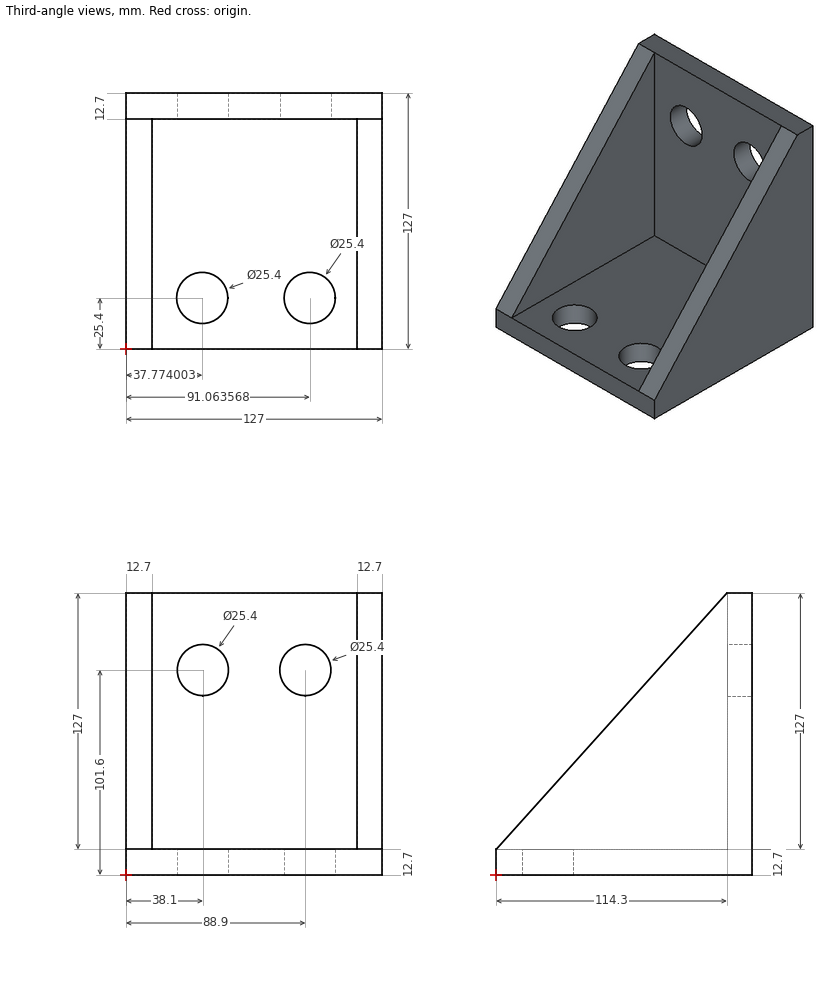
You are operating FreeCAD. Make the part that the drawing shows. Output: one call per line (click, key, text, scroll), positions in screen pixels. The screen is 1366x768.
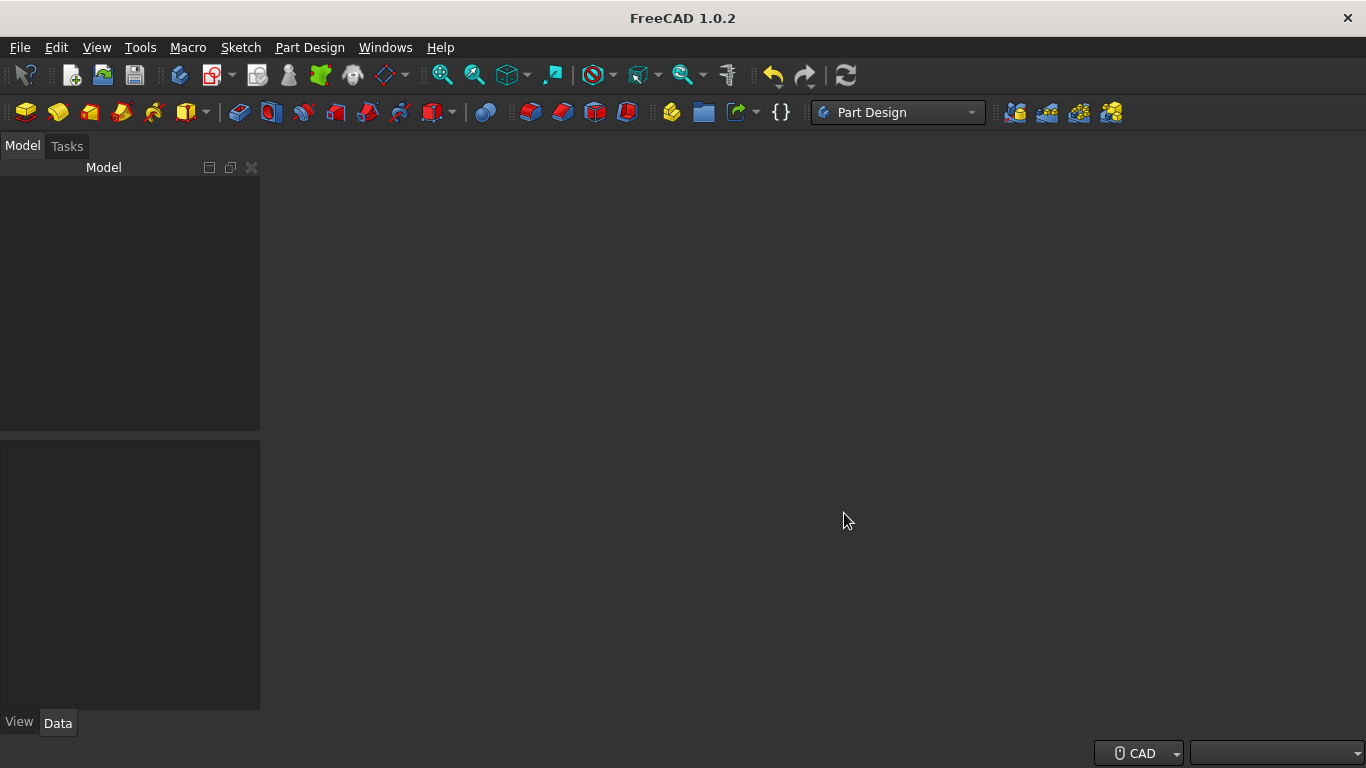
key(ctrl+n)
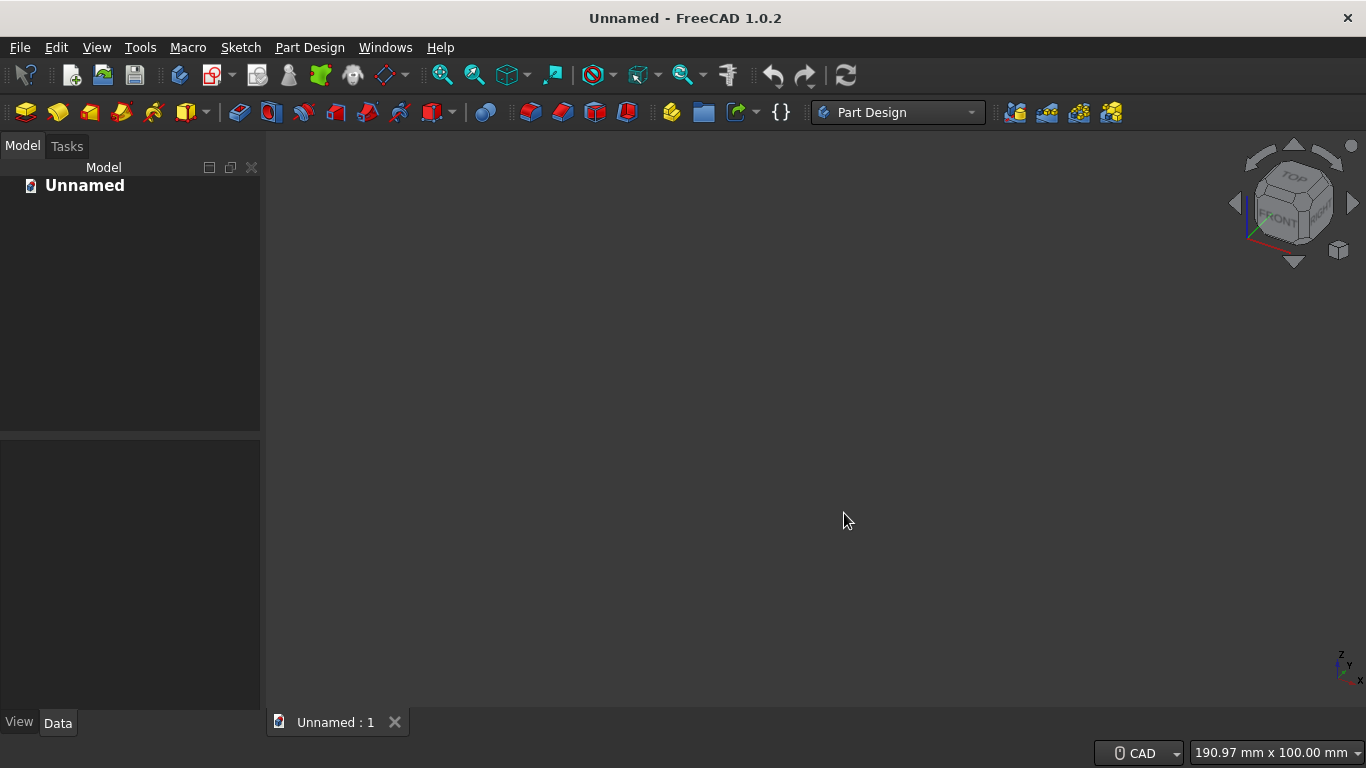
click(212, 76)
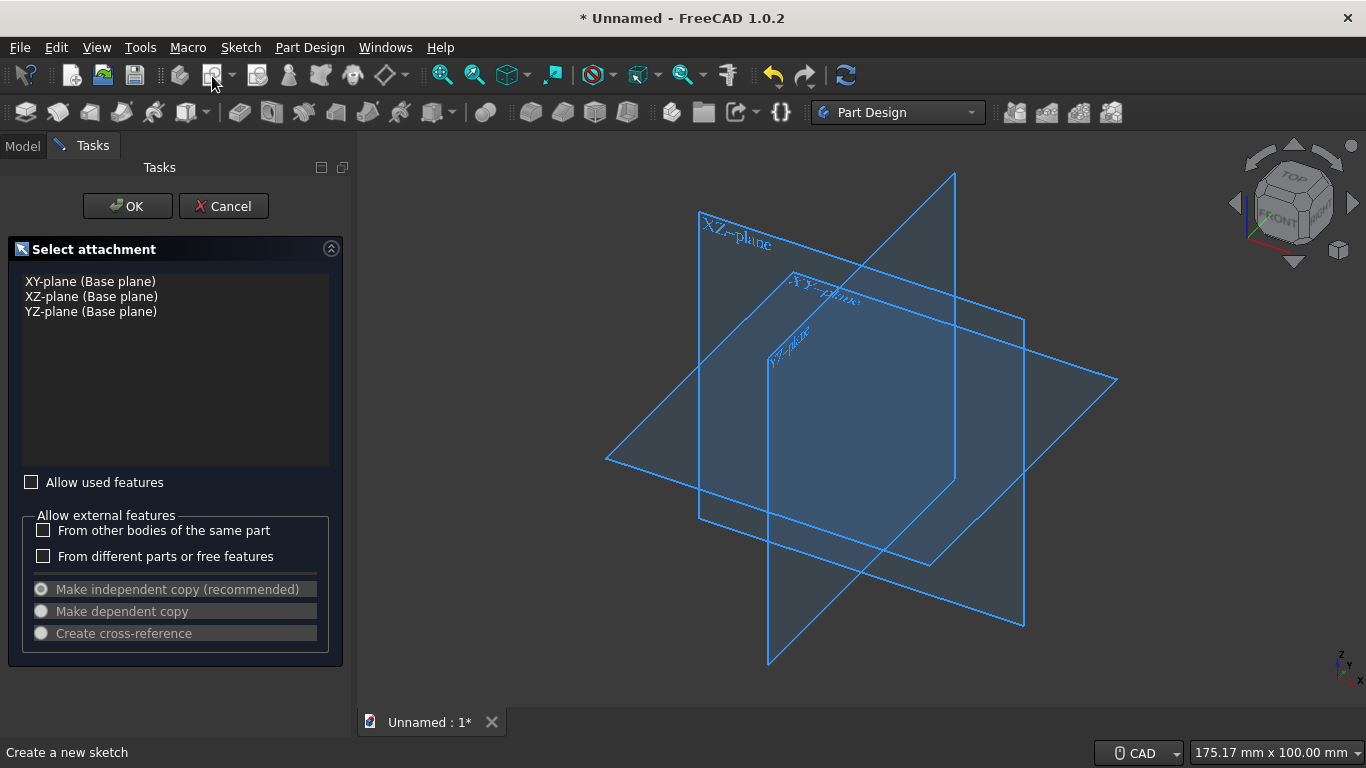
click(82, 282)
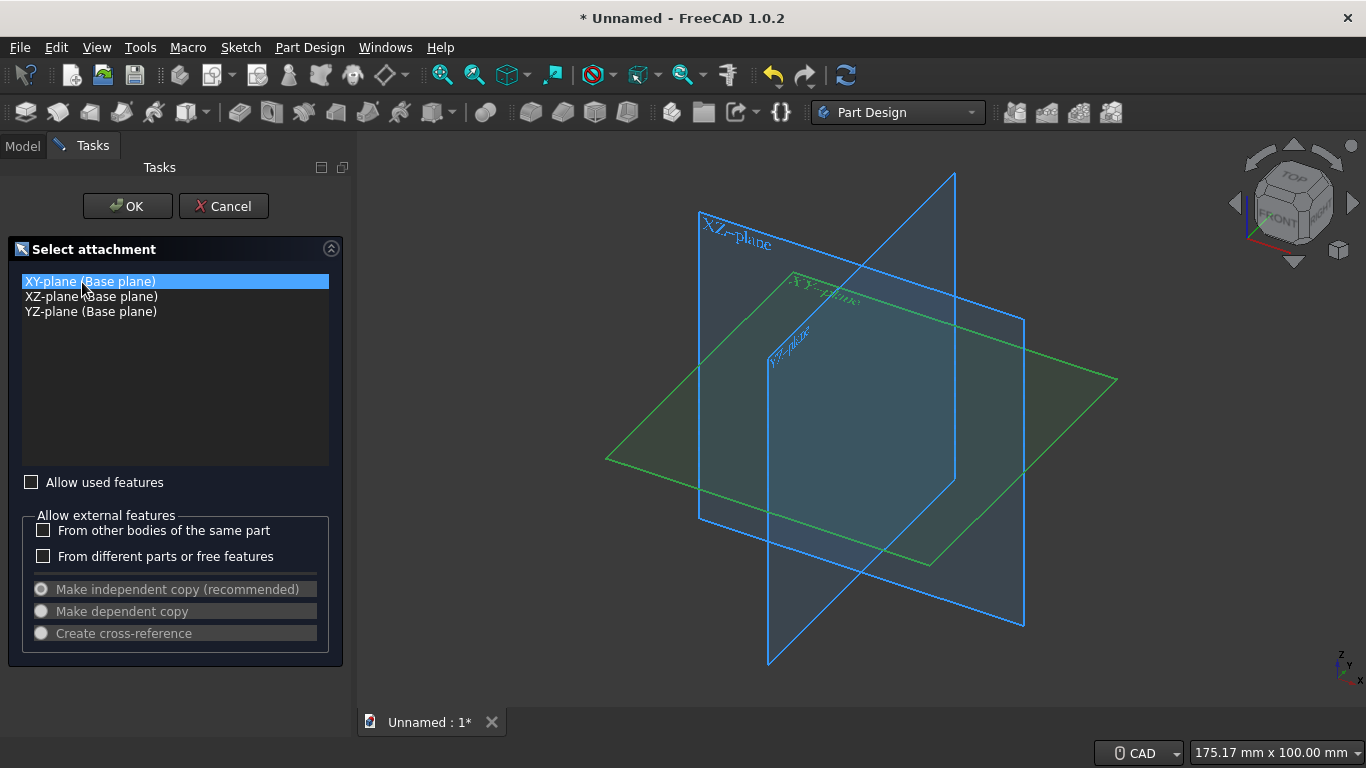
click(128, 206)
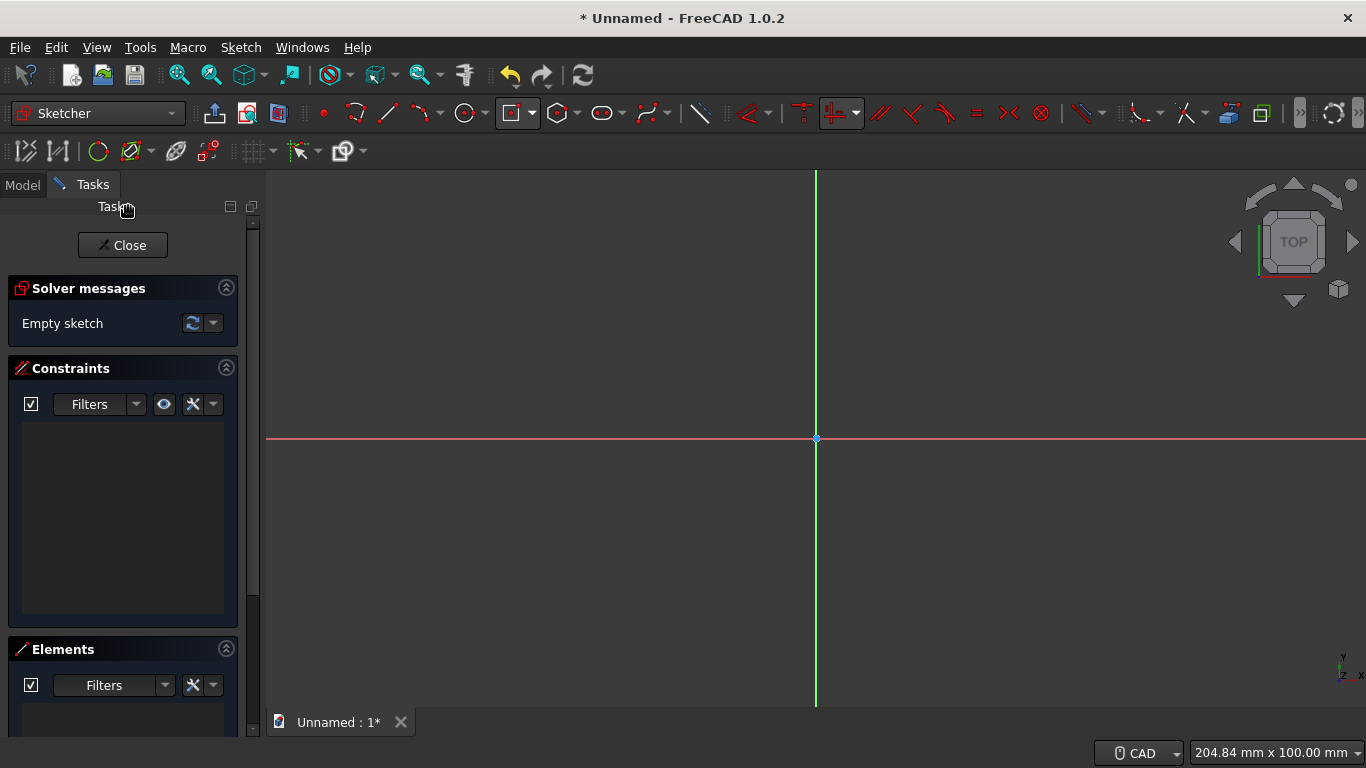
scroll(413, 679, down, 4)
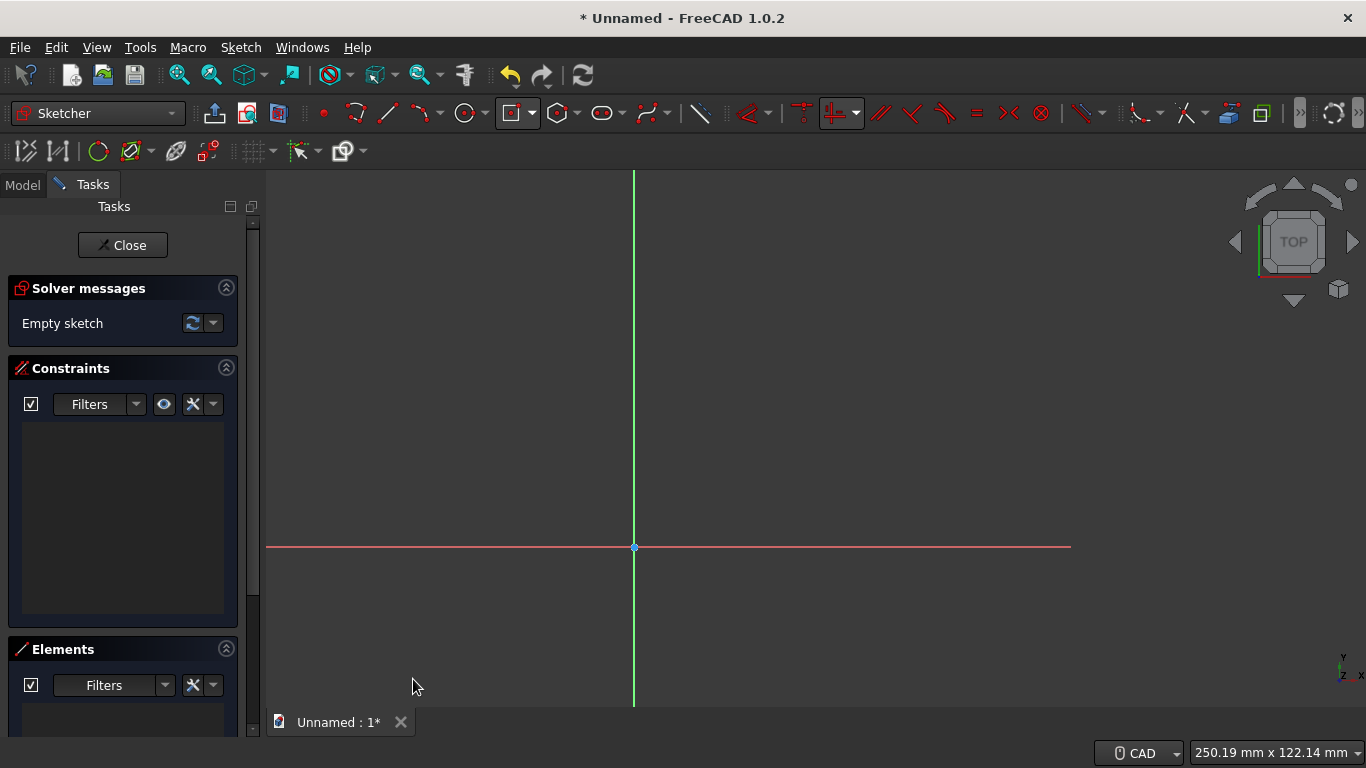
click(534, 114)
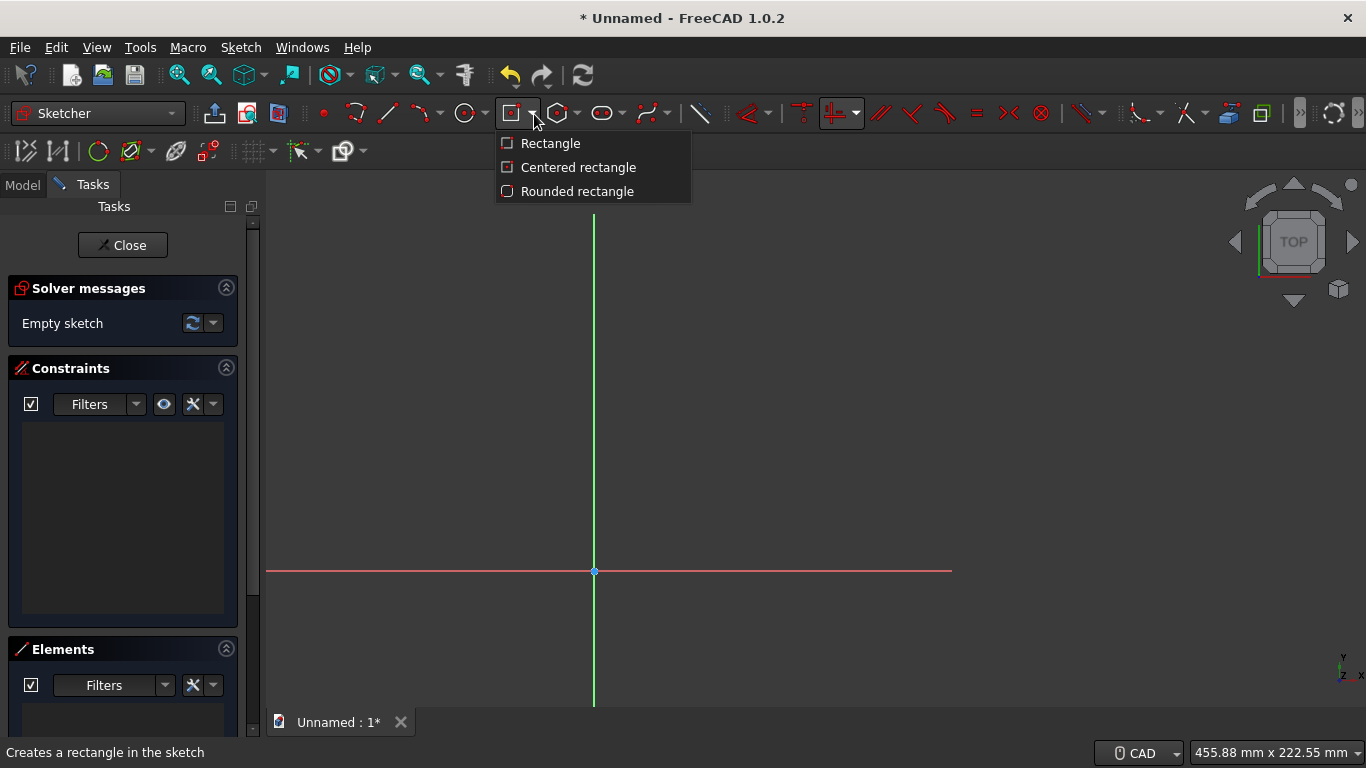
click(594, 143)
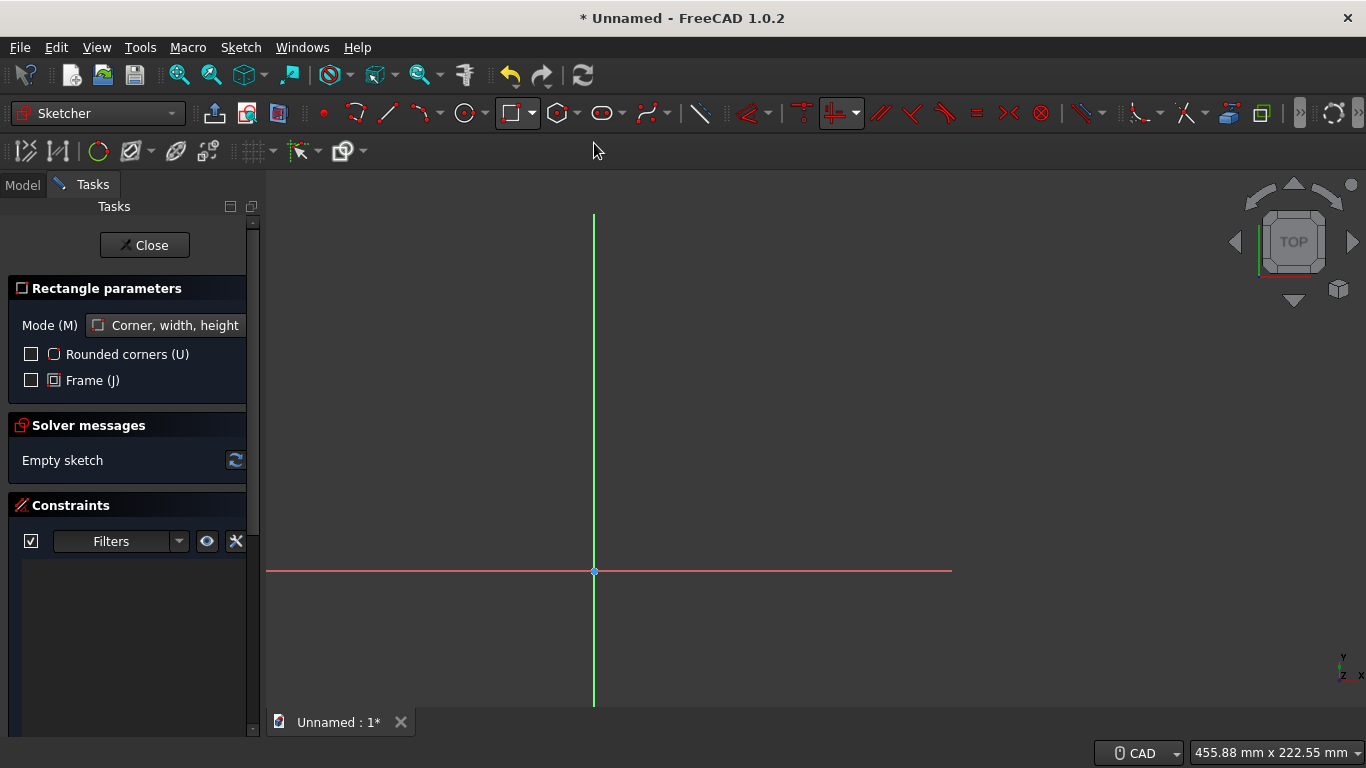
click(594, 571)
click(901, 265)
key(Escape)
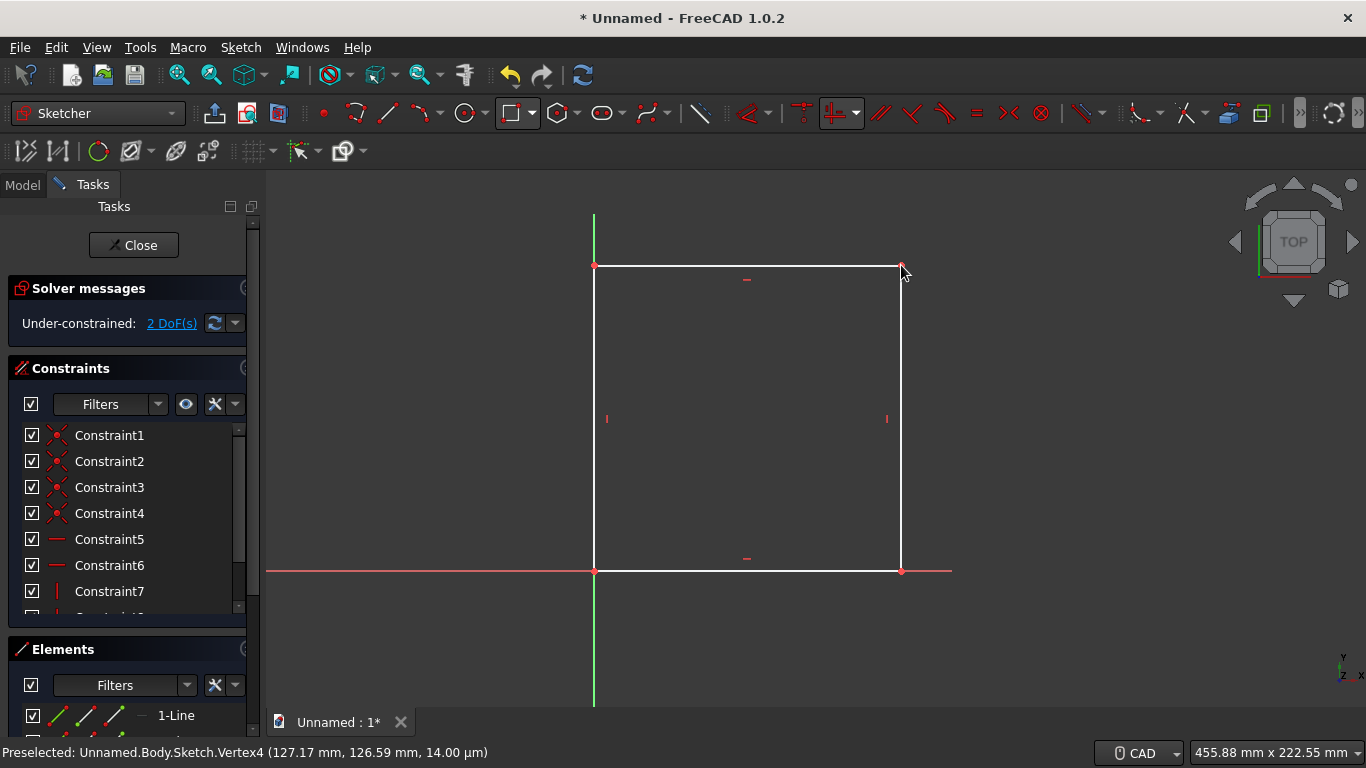
click(686, 571)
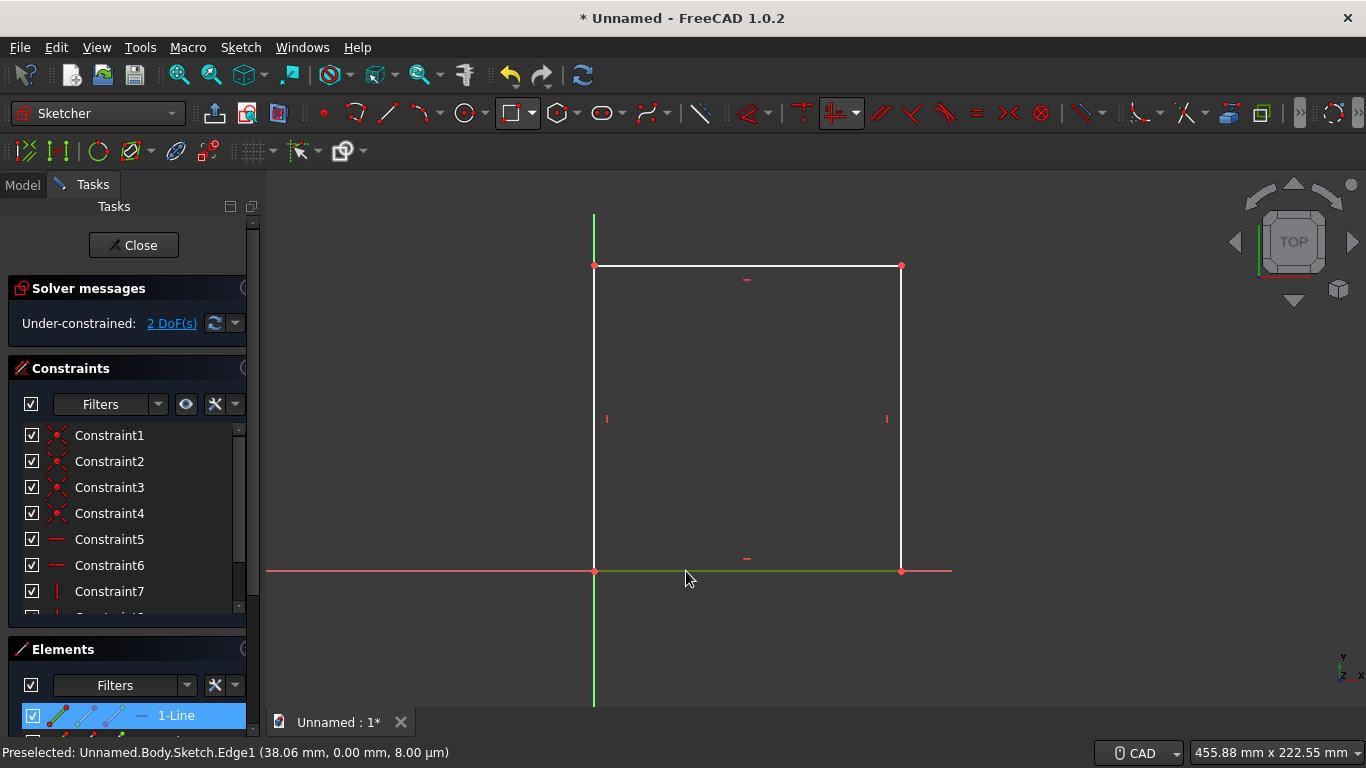
key(l)